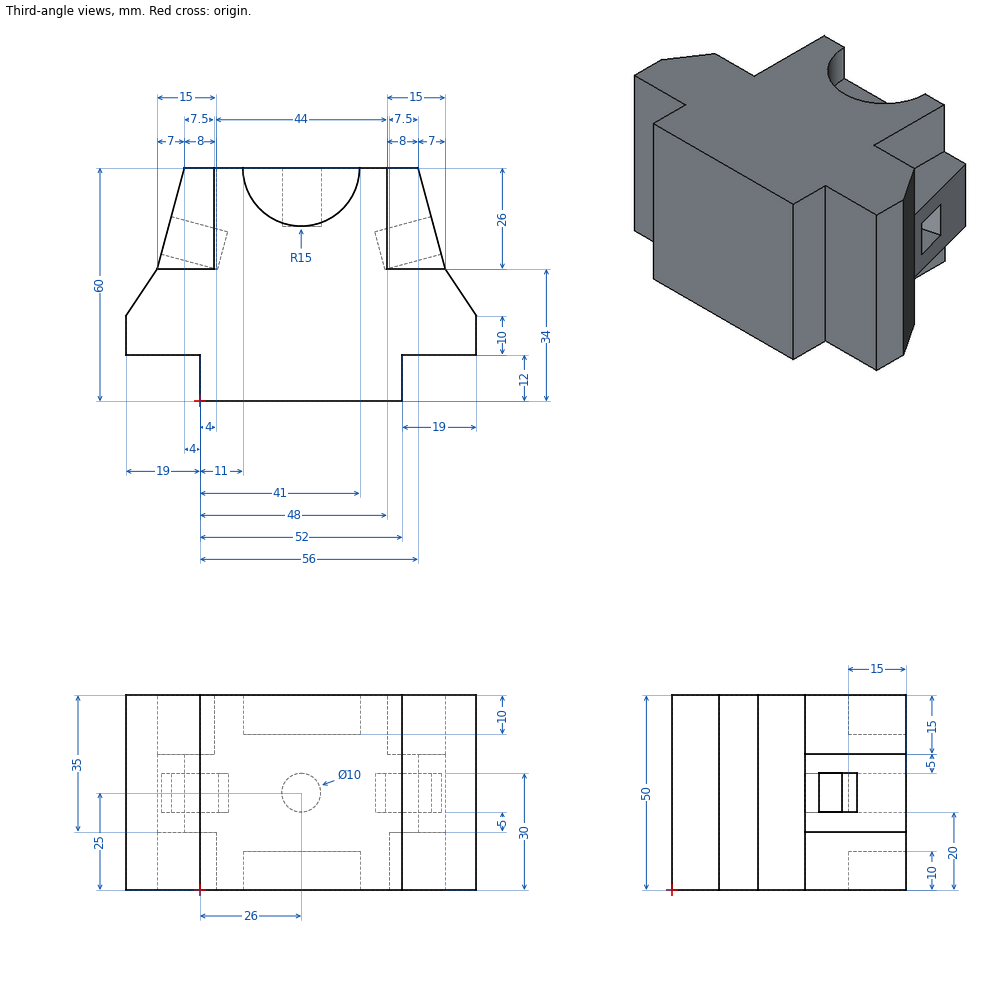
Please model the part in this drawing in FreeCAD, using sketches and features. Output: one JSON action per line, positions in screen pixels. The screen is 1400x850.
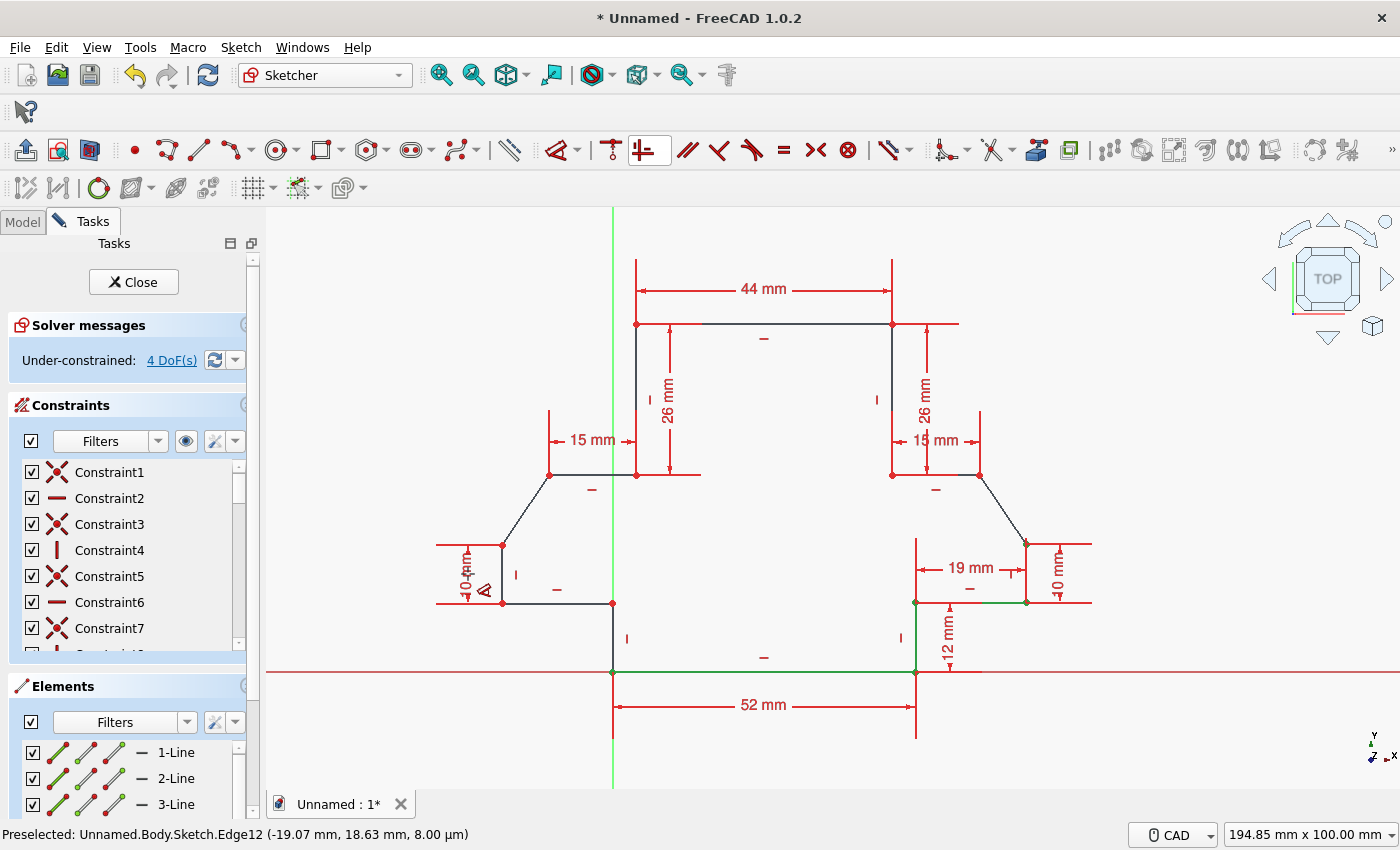
{"action": "left_click", "coordinate": [535, 604]}
{"action": "left_click", "coordinate": [557, 638]}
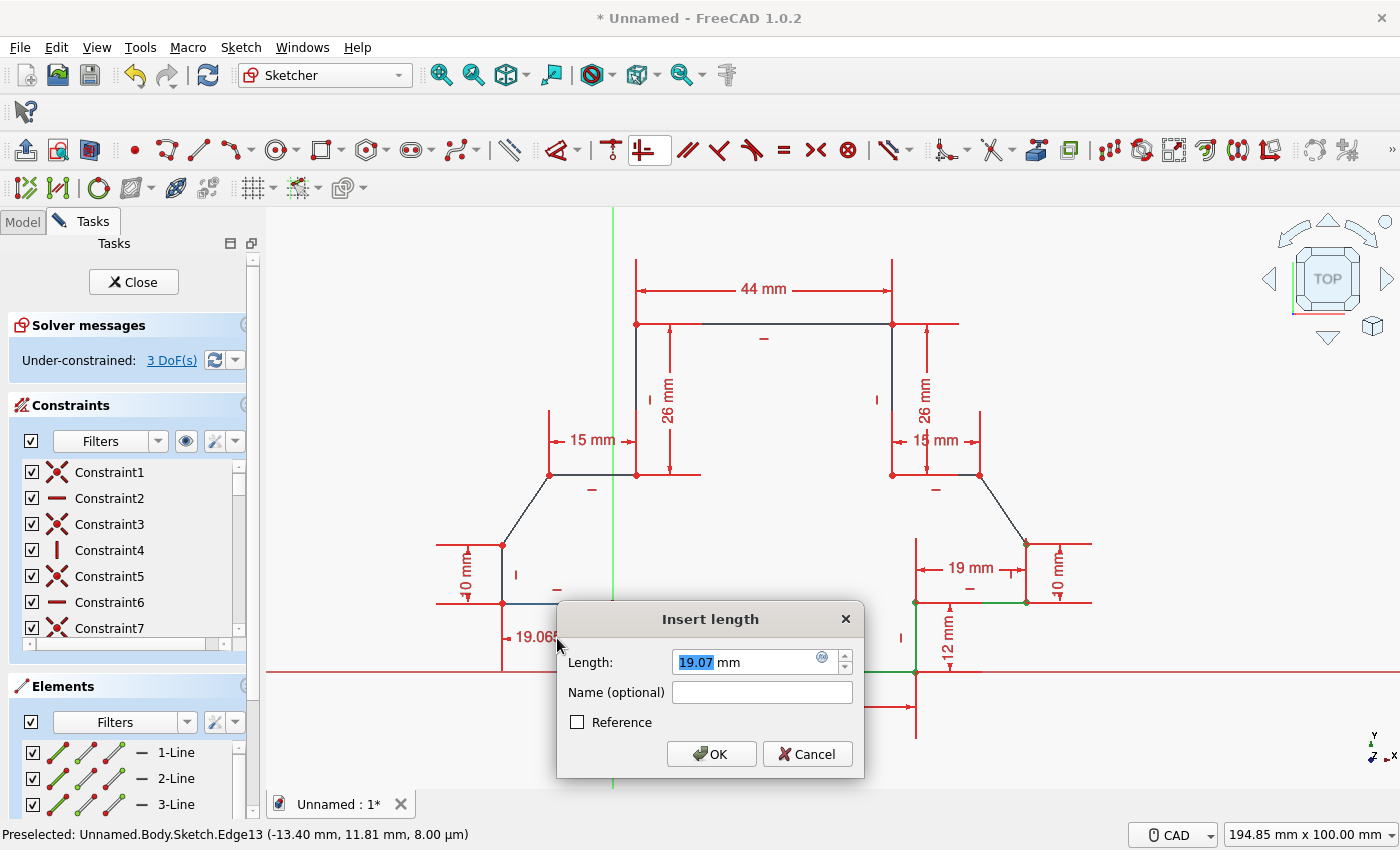
{"action": "type", "text": "19"}
{"action": "key", "text": "Return"}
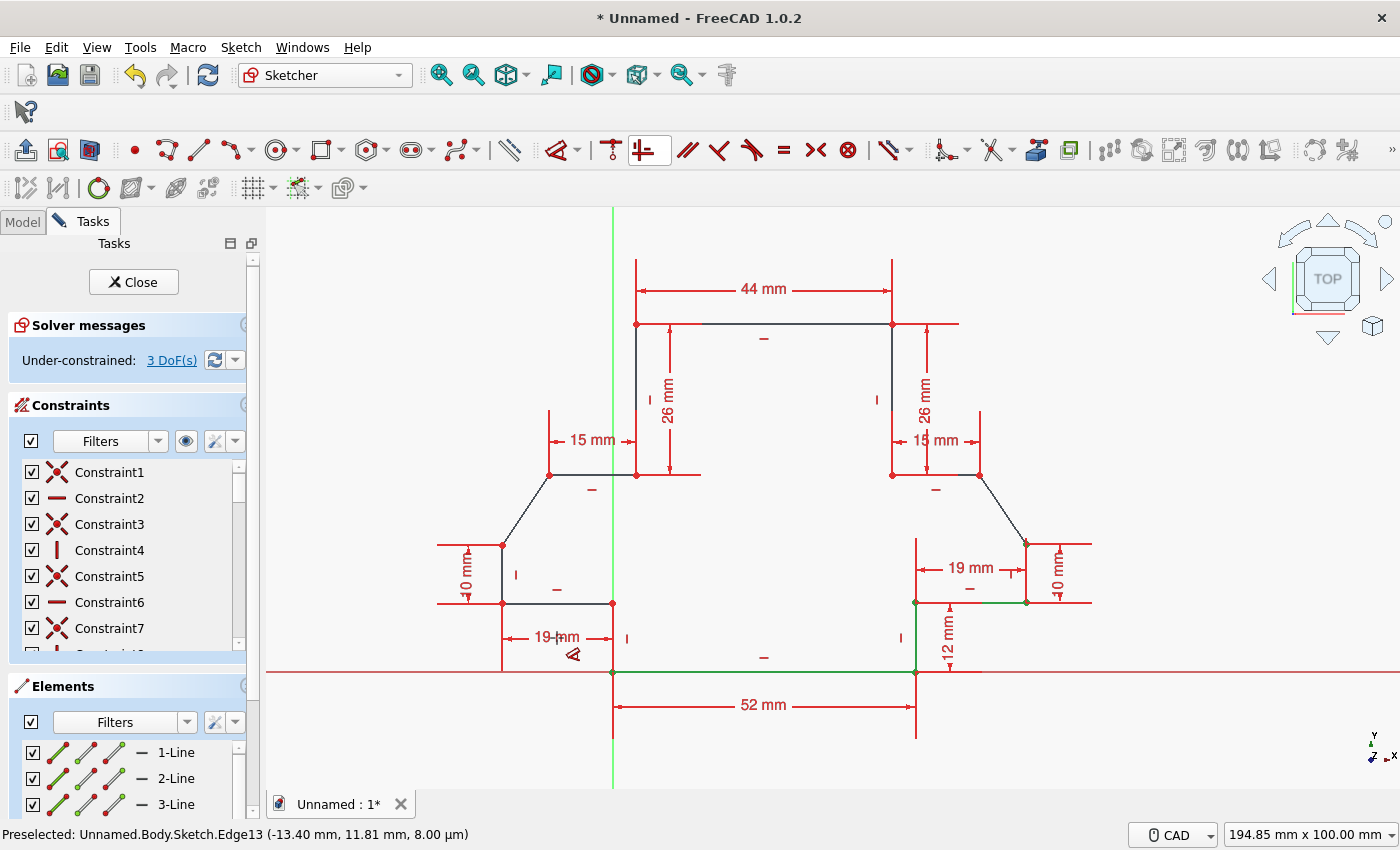
{"action": "left_click", "coordinate": [613, 624]}
{"action": "left_click", "coordinate": [647, 638]}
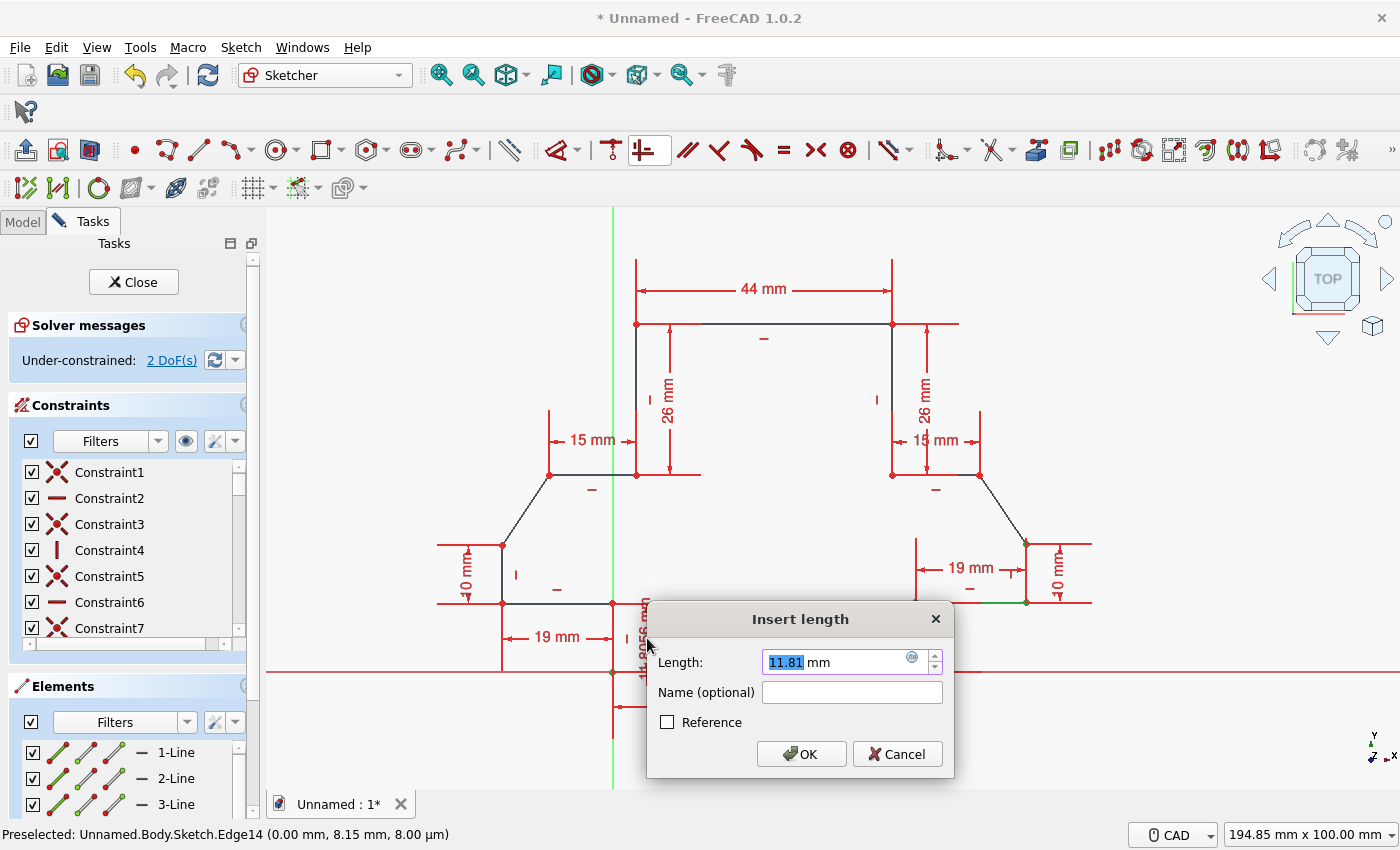
{"action": "type", "text": "12"}
{"action": "key", "text": "Return"}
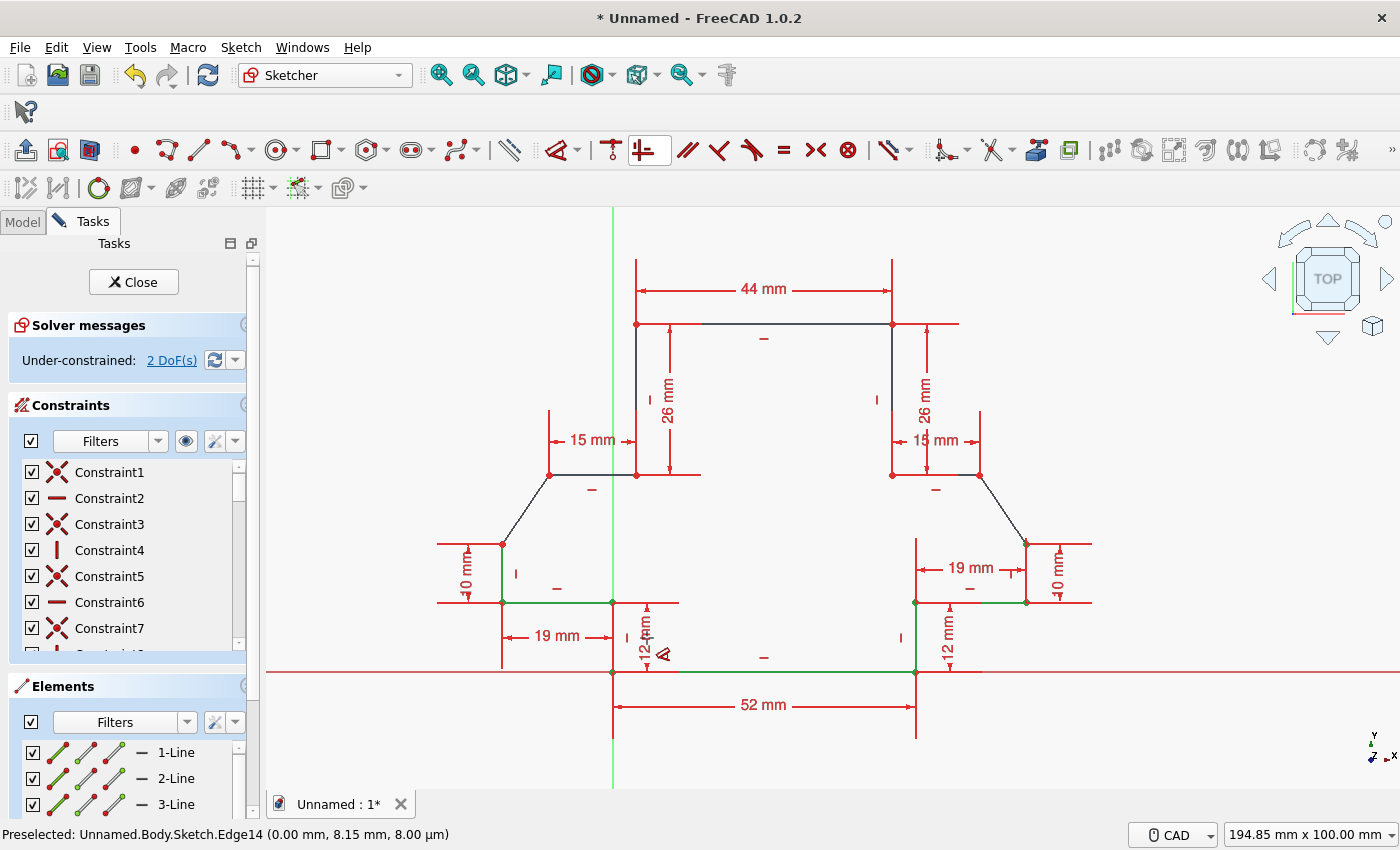
{"action": "scroll", "coordinate": [636, 324], "scroll_direction": "up", "scroll_amount": 3}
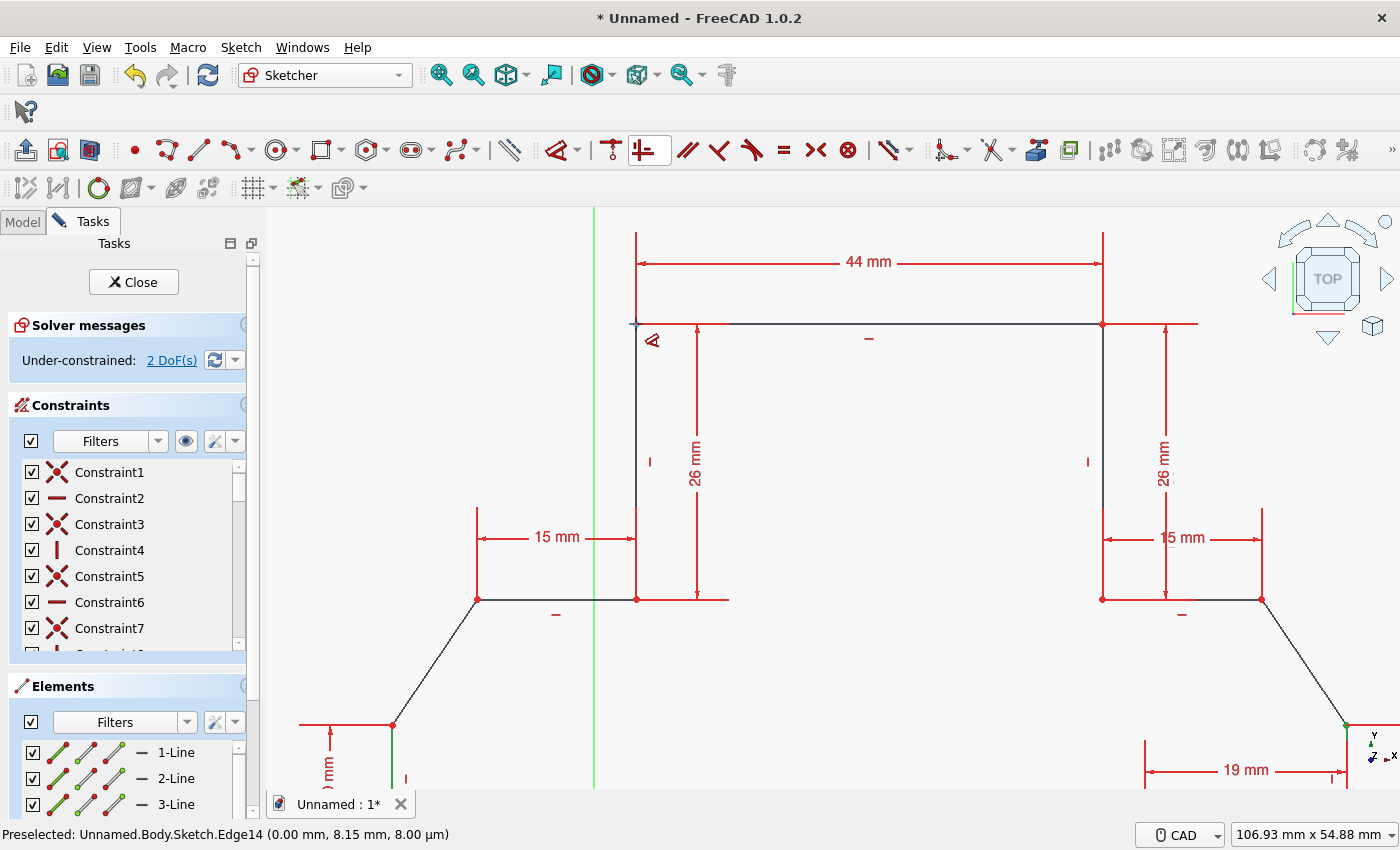
{"action": "left_click", "coordinate": [636, 324]}
{"action": "left_click", "coordinate": [615, 290]}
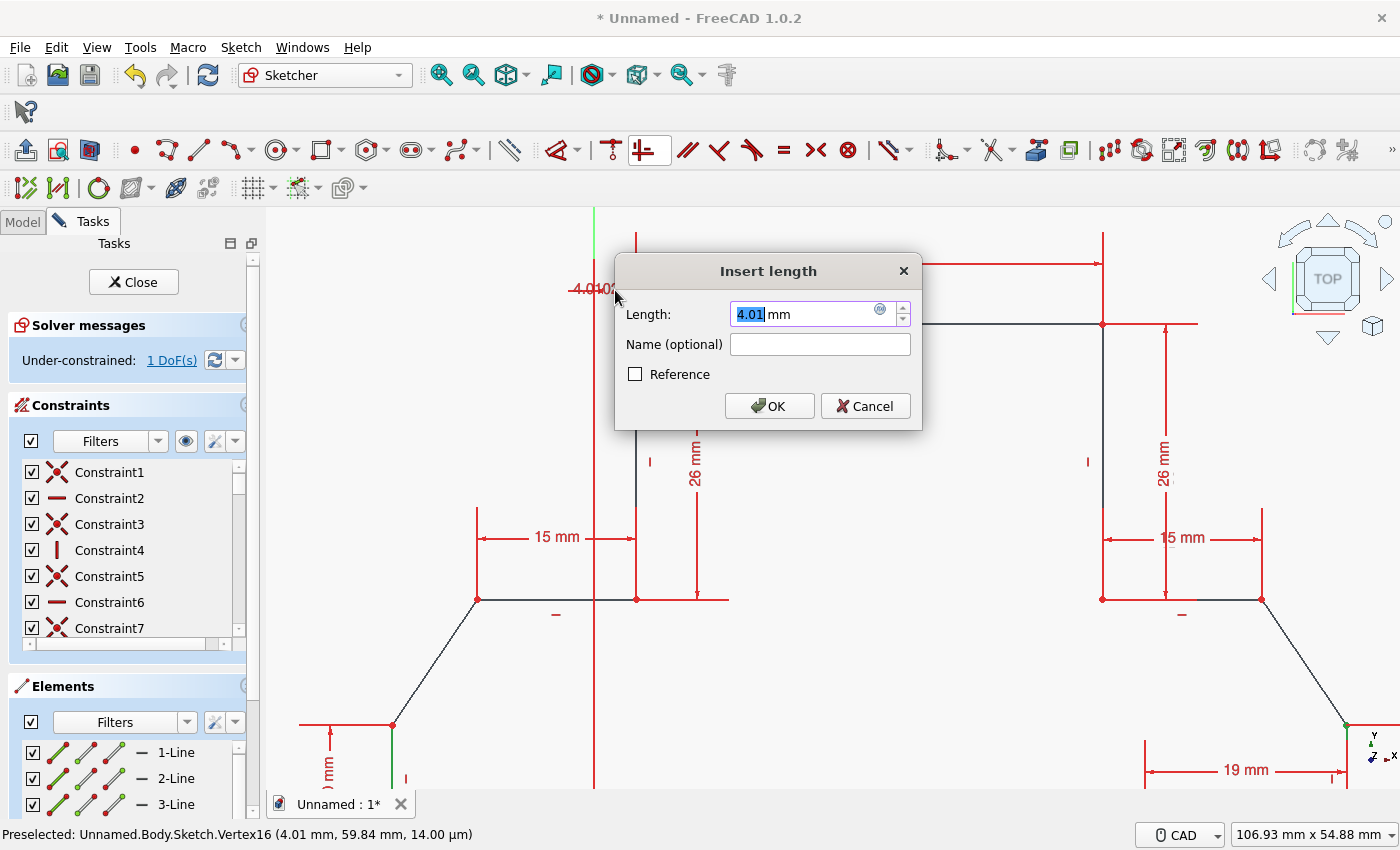
{"action": "type", "text": "4"}
{"action": "key", "text": "Return"}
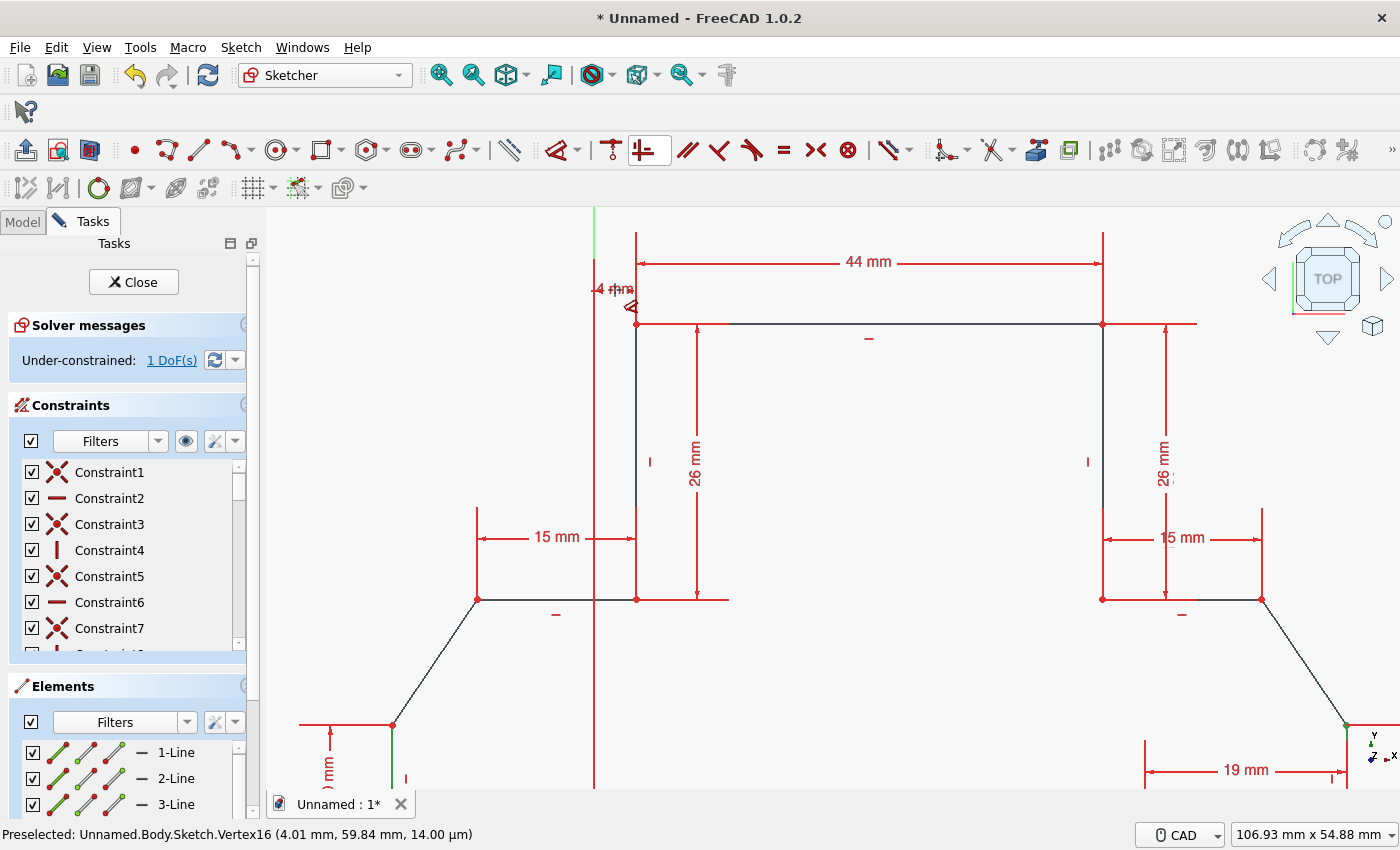
{"action": "scroll", "coordinate": [637, 325], "scroll_direction": "down", "scroll_amount": 3}